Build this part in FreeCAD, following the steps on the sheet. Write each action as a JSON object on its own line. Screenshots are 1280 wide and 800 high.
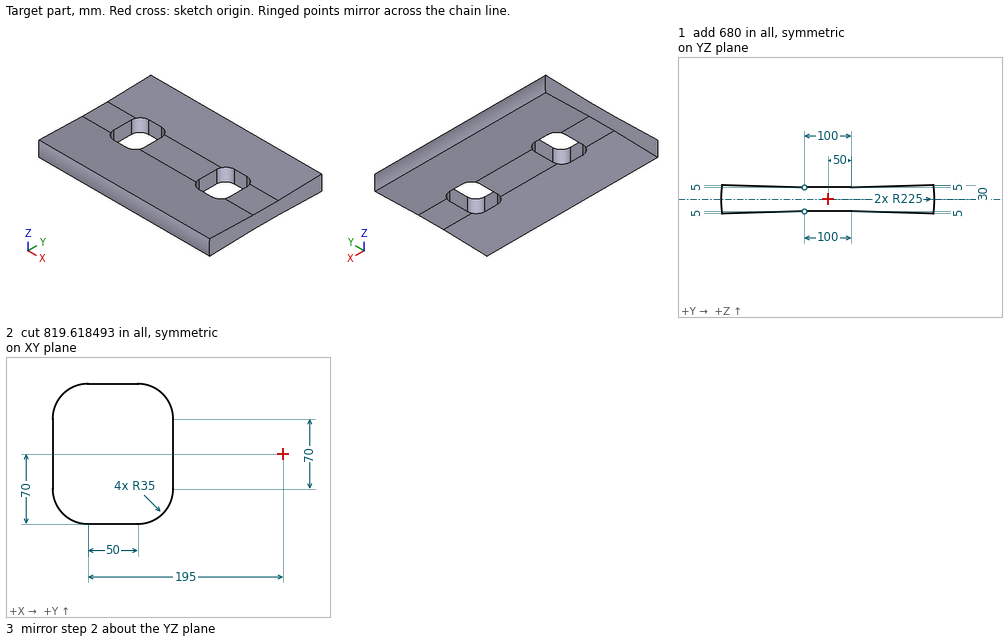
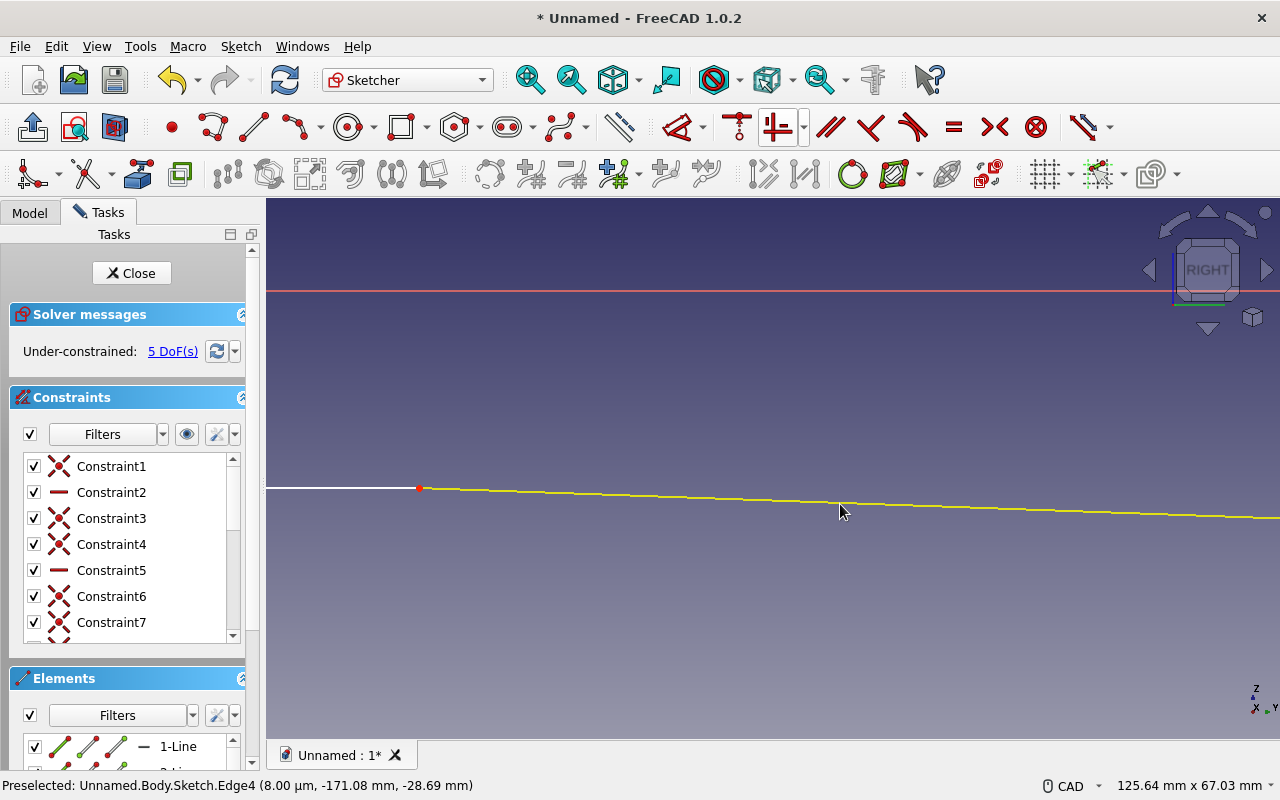
{"action": "left_click", "coordinate": [839, 503]}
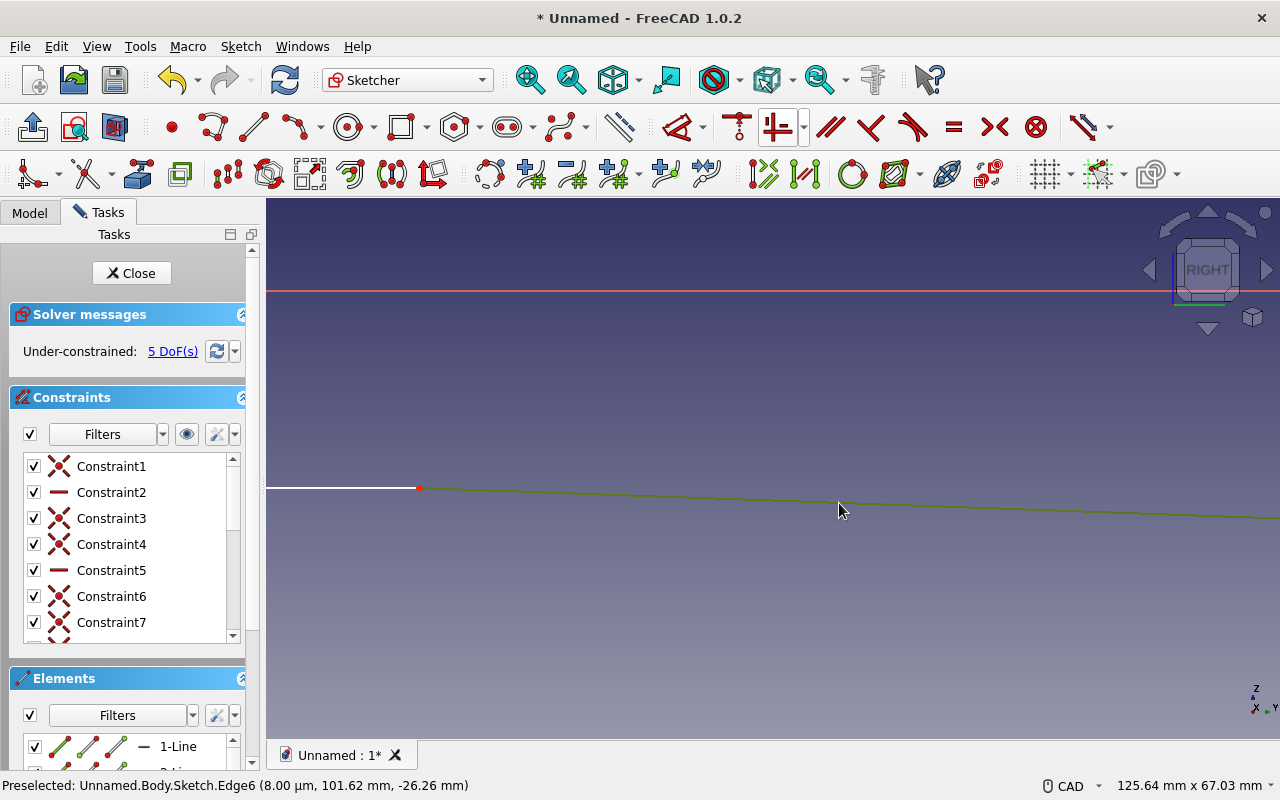
{"action": "key", "text": "i"}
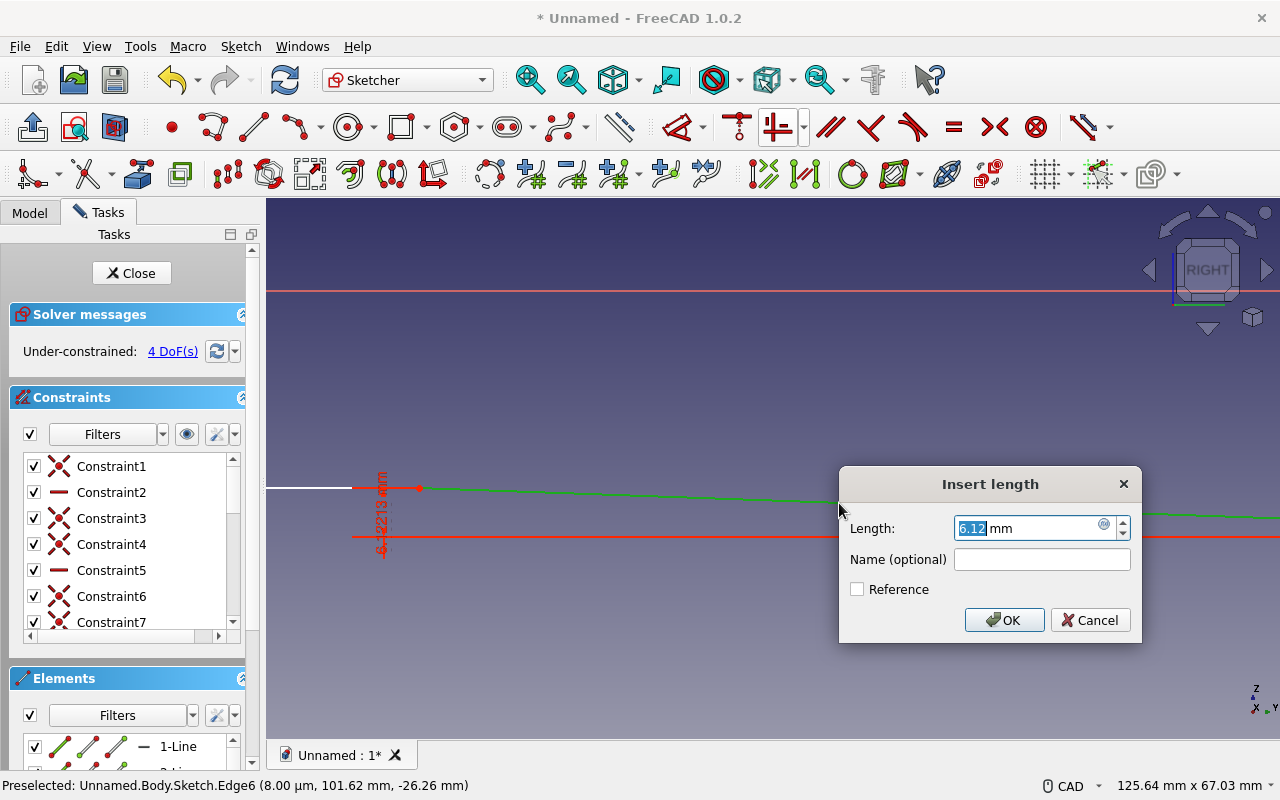
{"action": "type", "text": "5"}
{"action": "key", "text": "Return"}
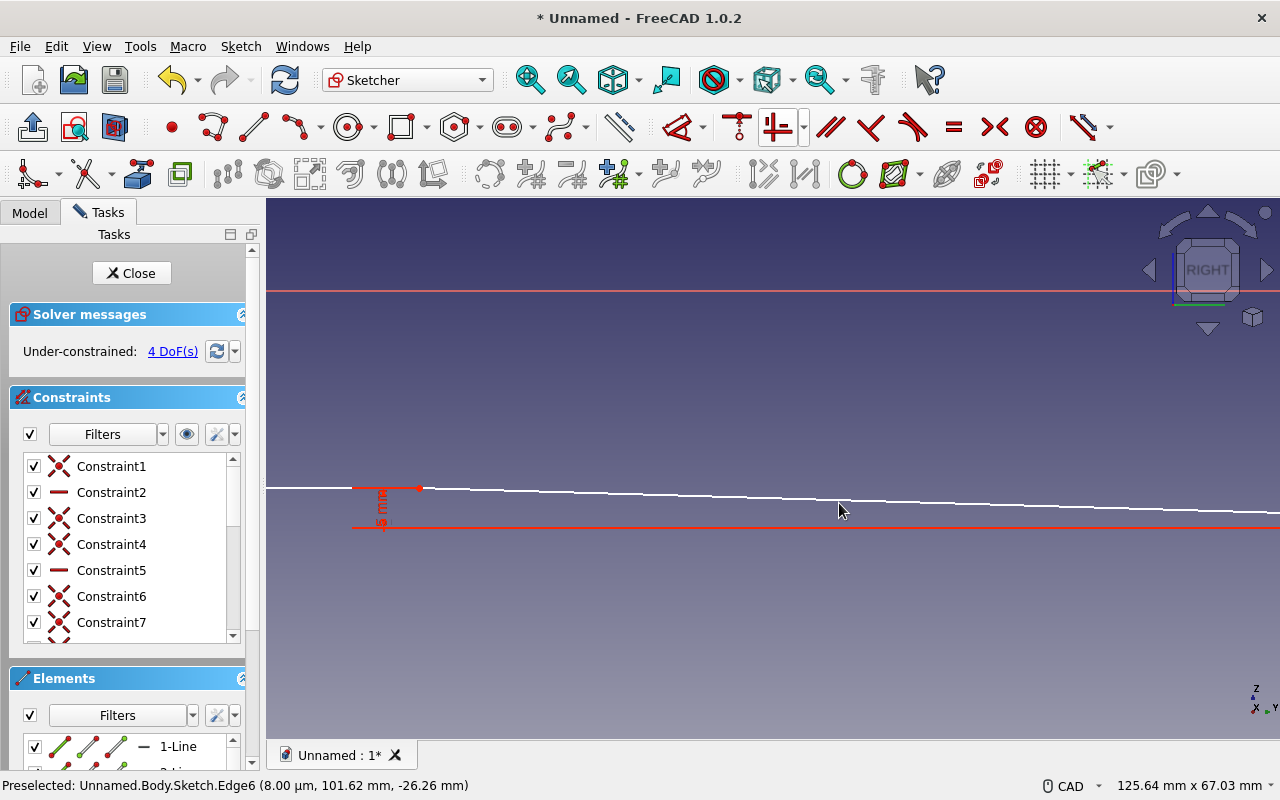
{"action": "scroll", "coordinate": [840, 504], "scroll_direction": "down", "scroll_amount": 9}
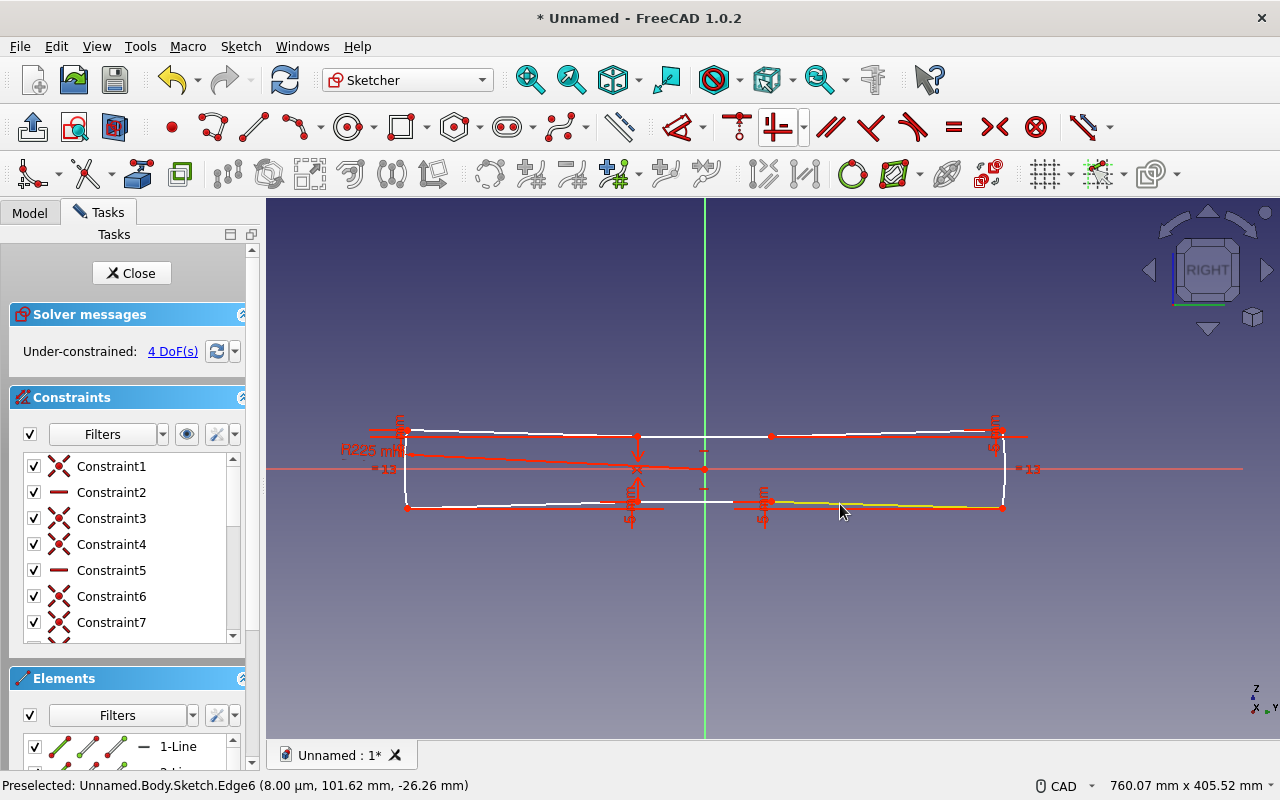
{"action": "left_click", "coordinate": [731, 437]}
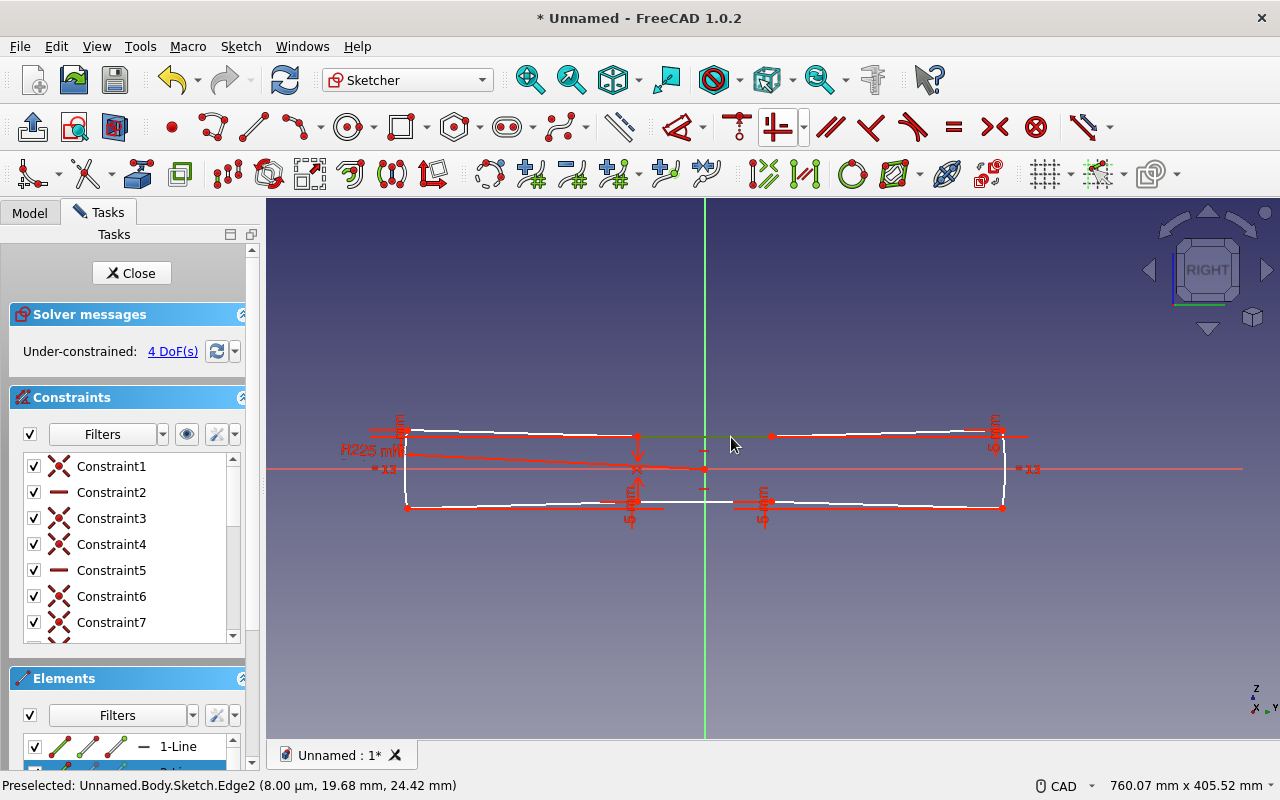
{"action": "key", "text": "l"}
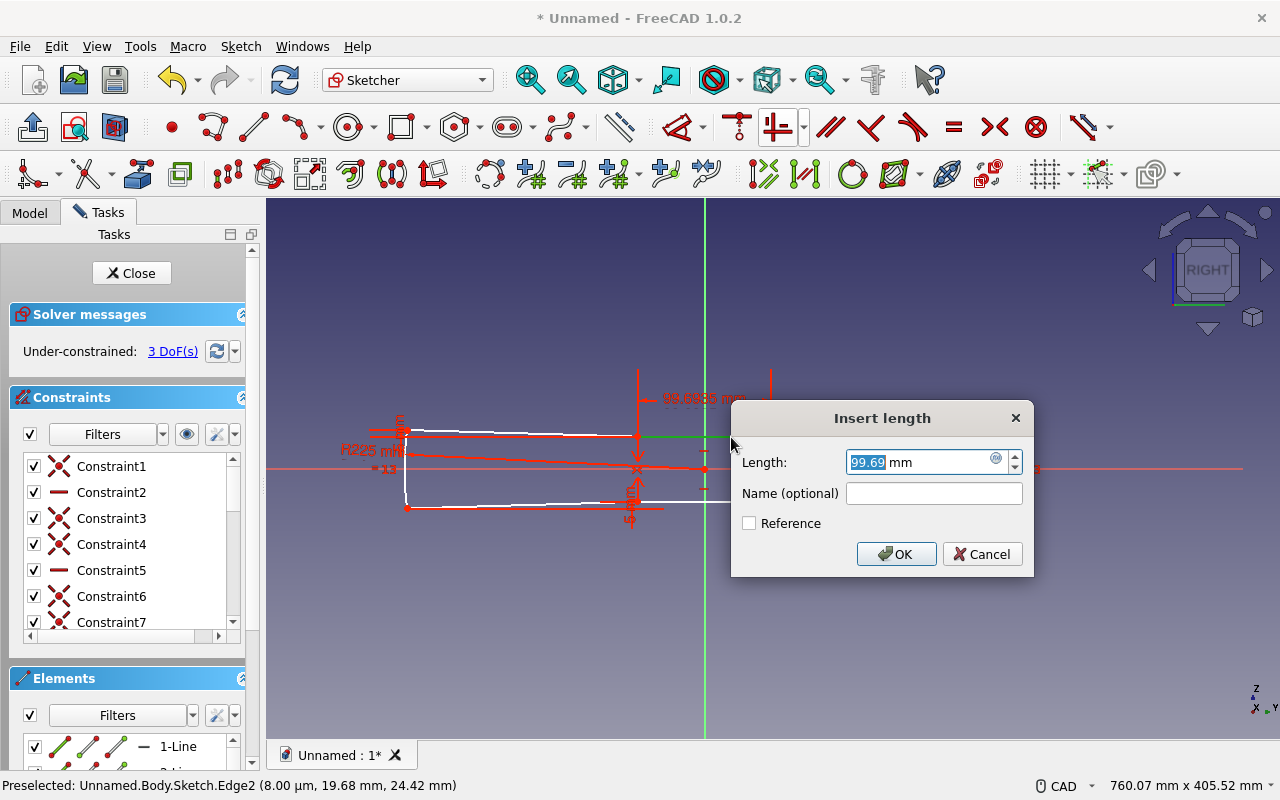
{"action": "type", "text": "100"}
{"action": "key", "text": "Return"}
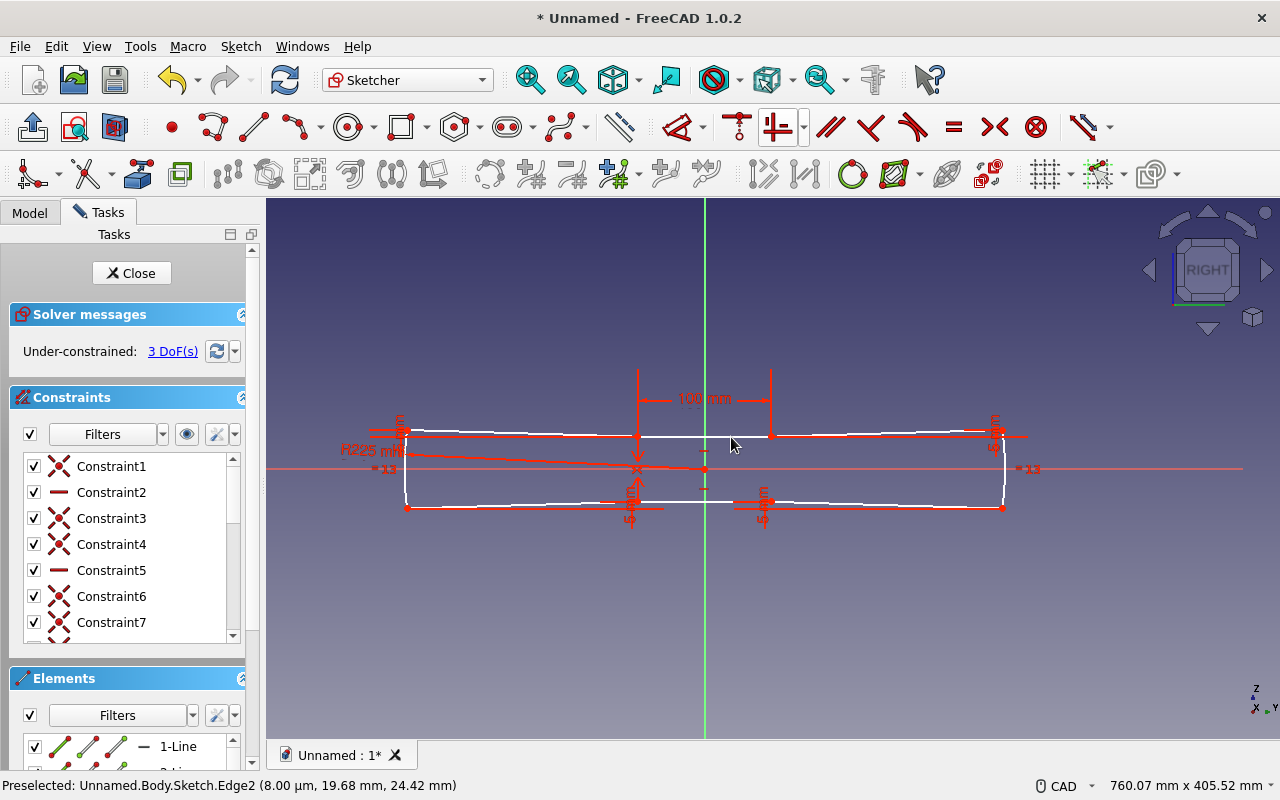
{"action": "left_click", "coordinate": [678, 502]}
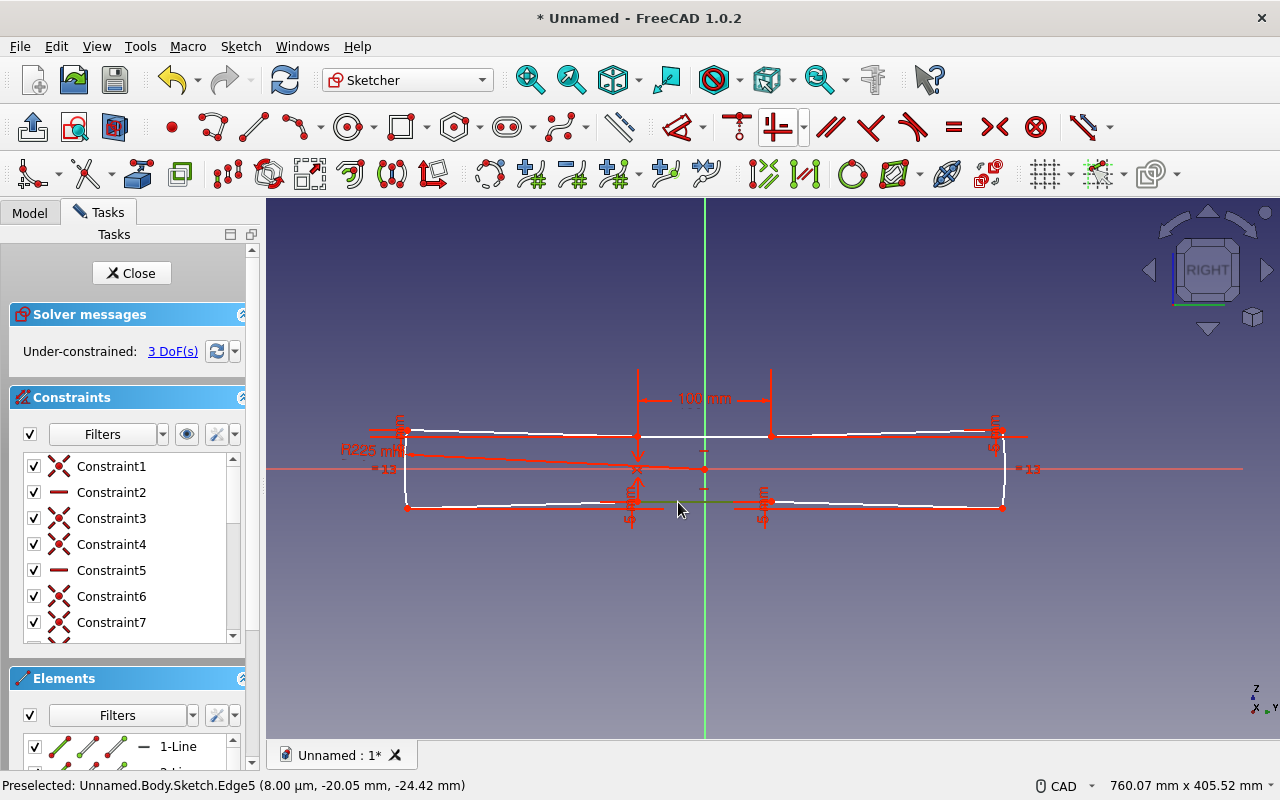
{"action": "key", "text": "l"}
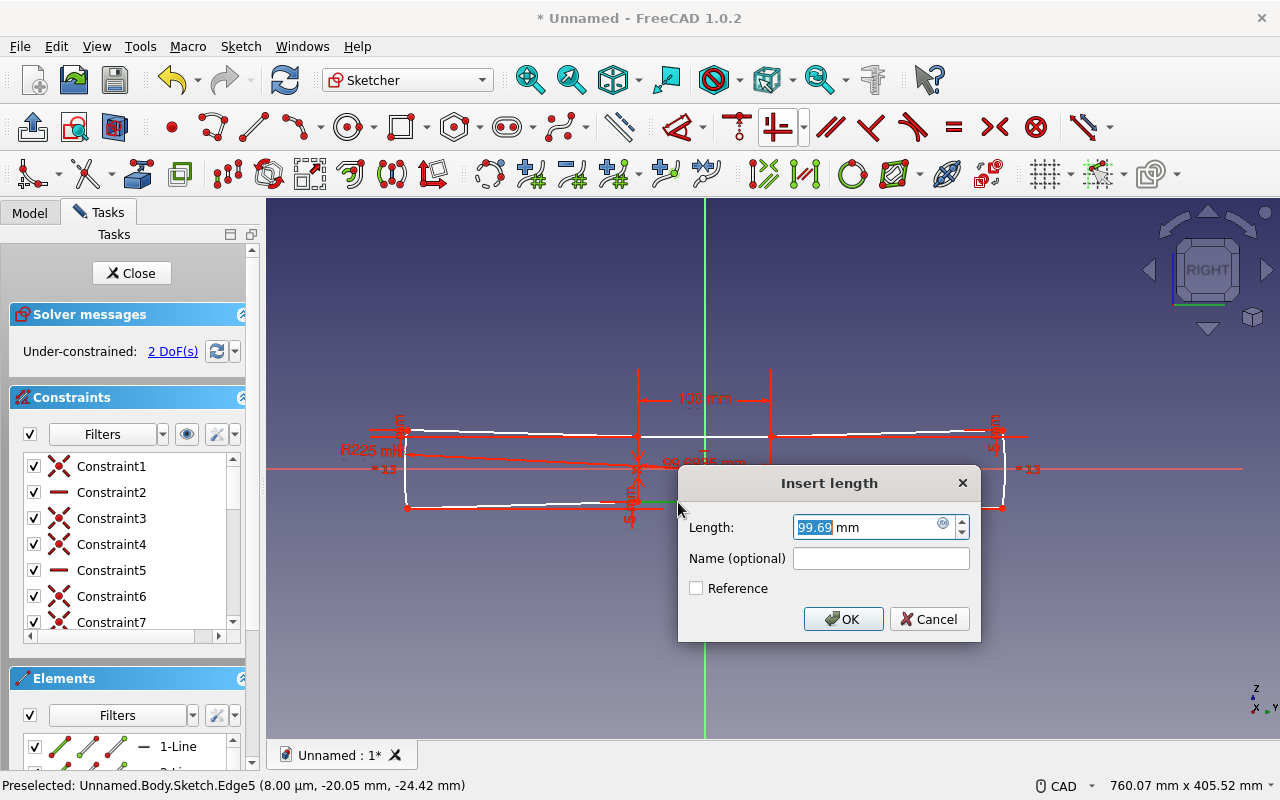
{"action": "type", "text": "100"}
{"action": "key", "text": "Return"}